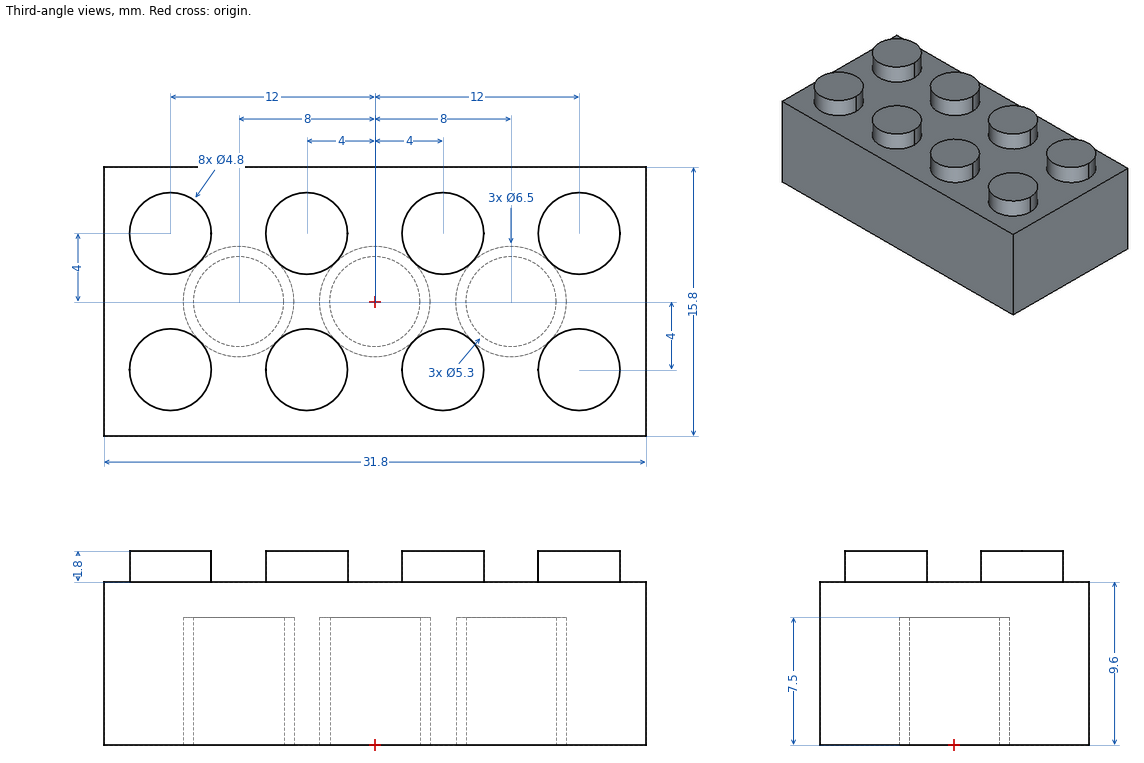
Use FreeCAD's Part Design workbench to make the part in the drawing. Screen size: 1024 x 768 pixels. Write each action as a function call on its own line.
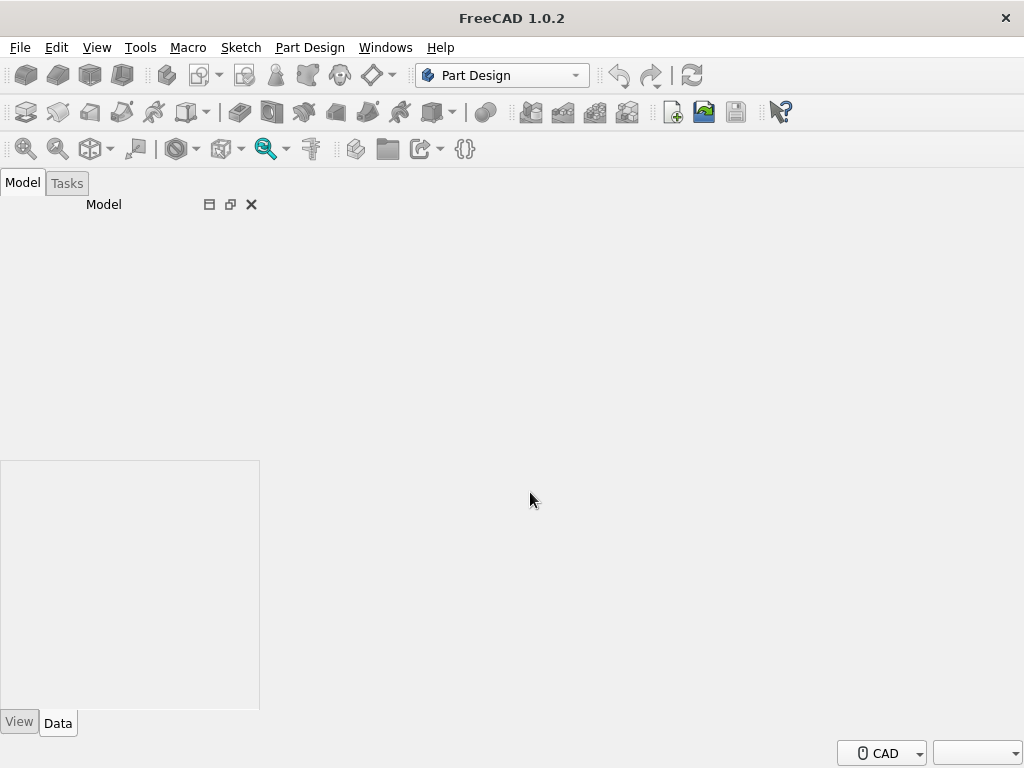
click(672, 112)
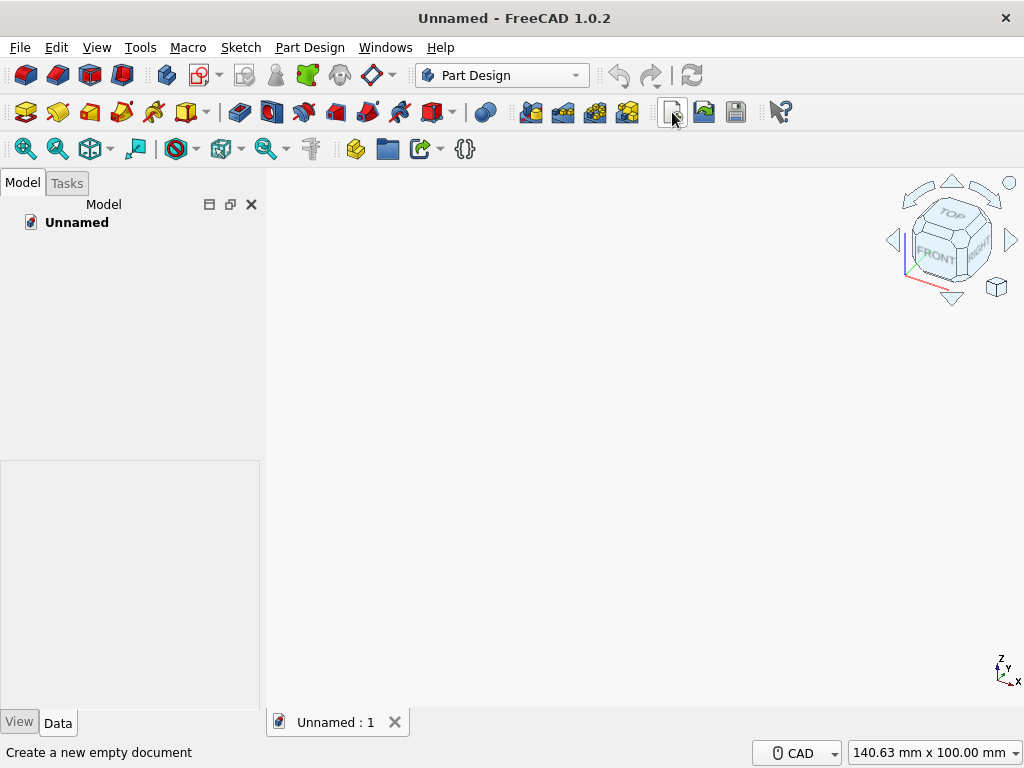
click(200, 76)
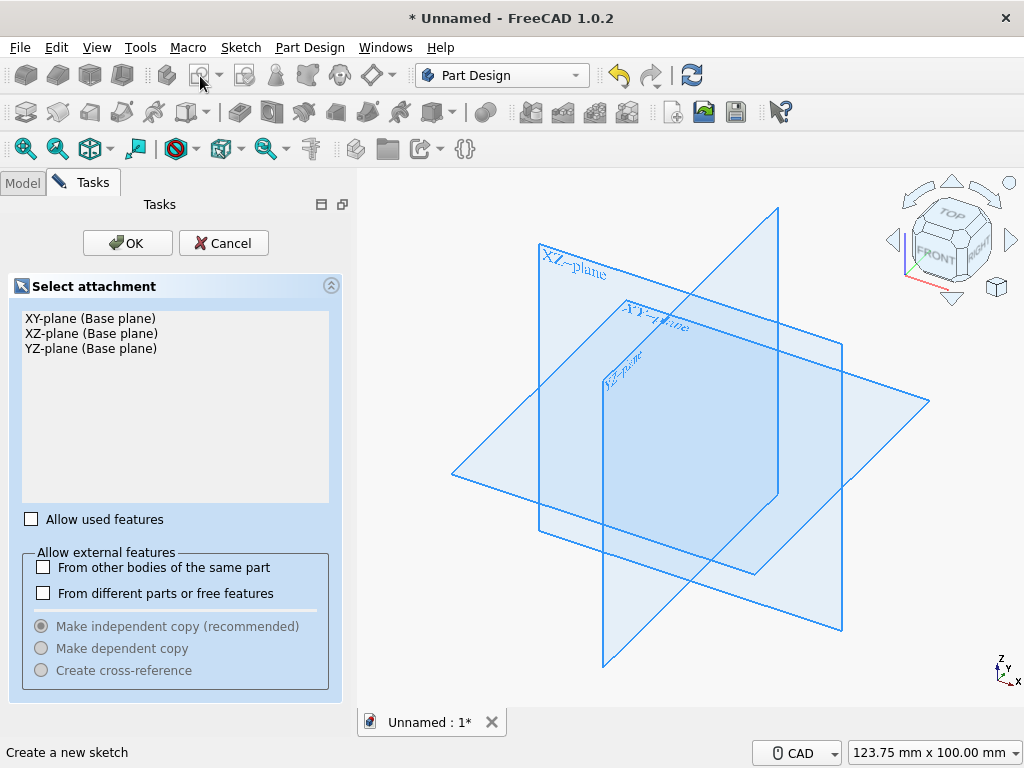
click(82, 318)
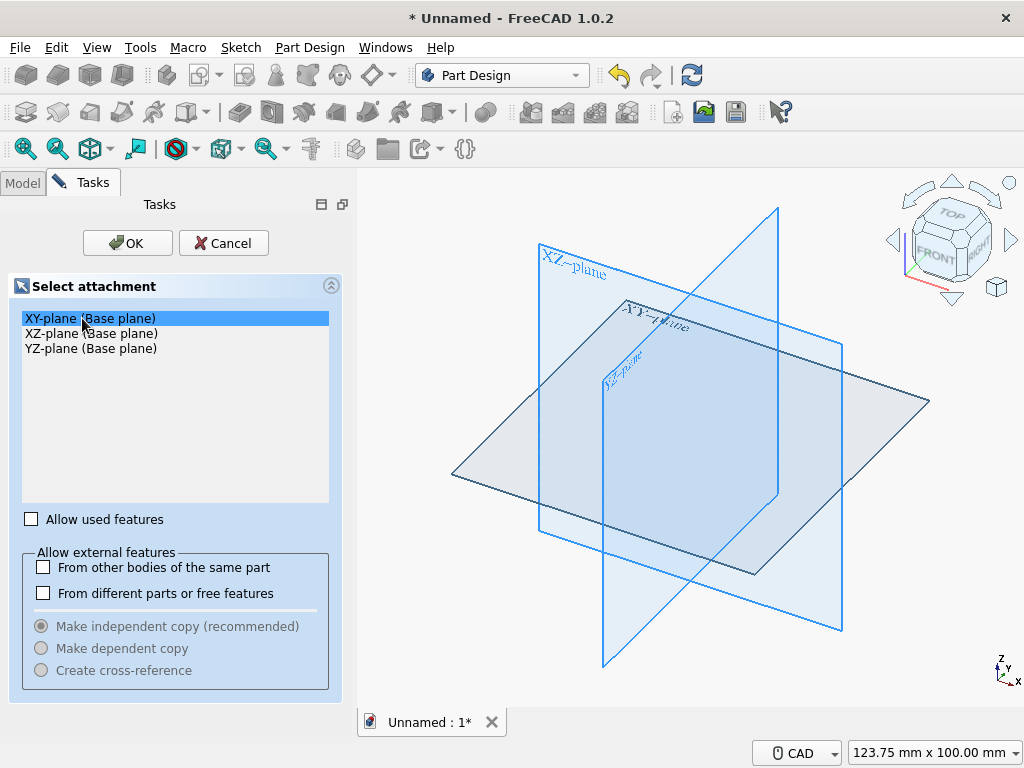
click(128, 243)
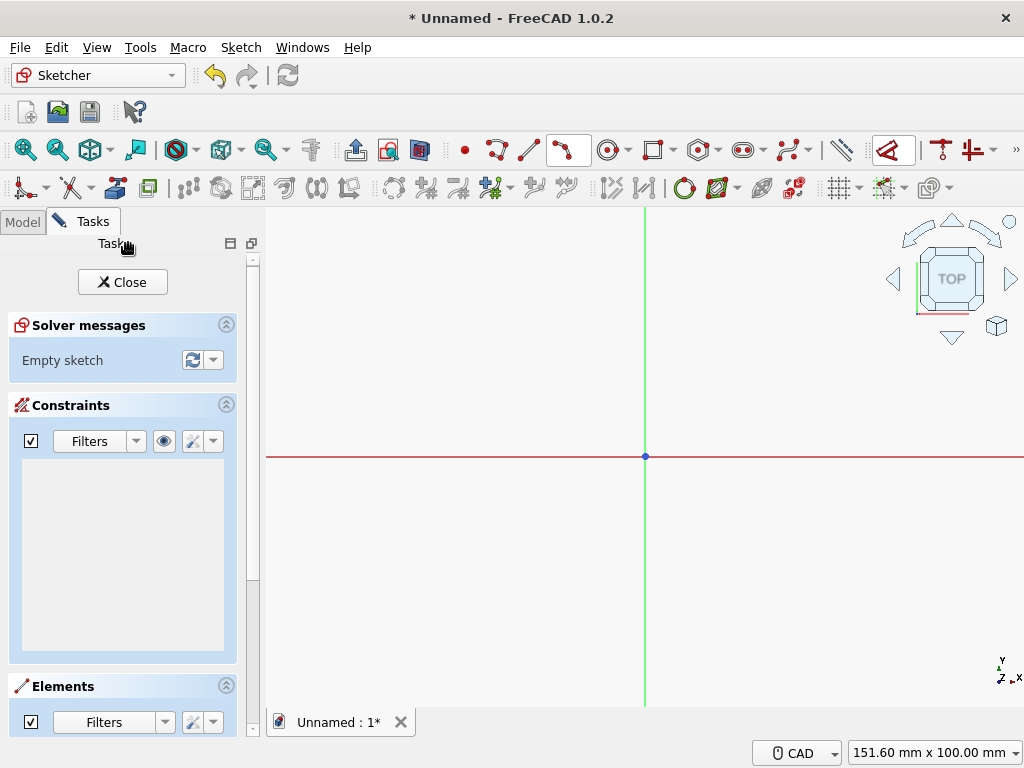
scroll(685, 457, up, 5)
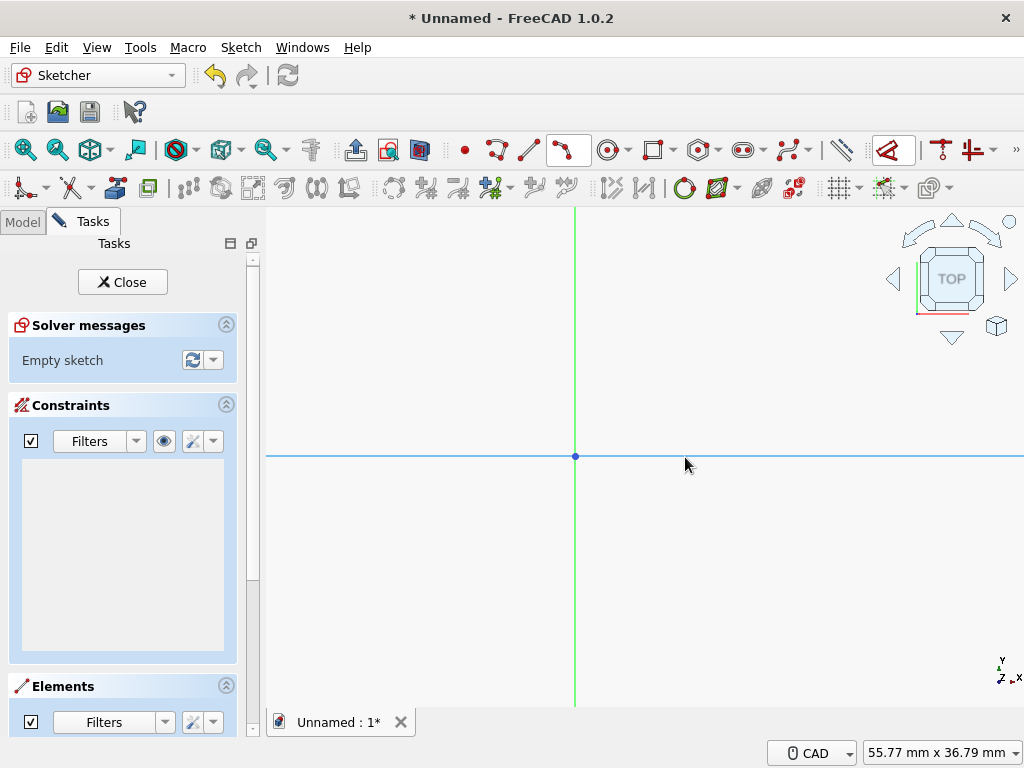
click(676, 150)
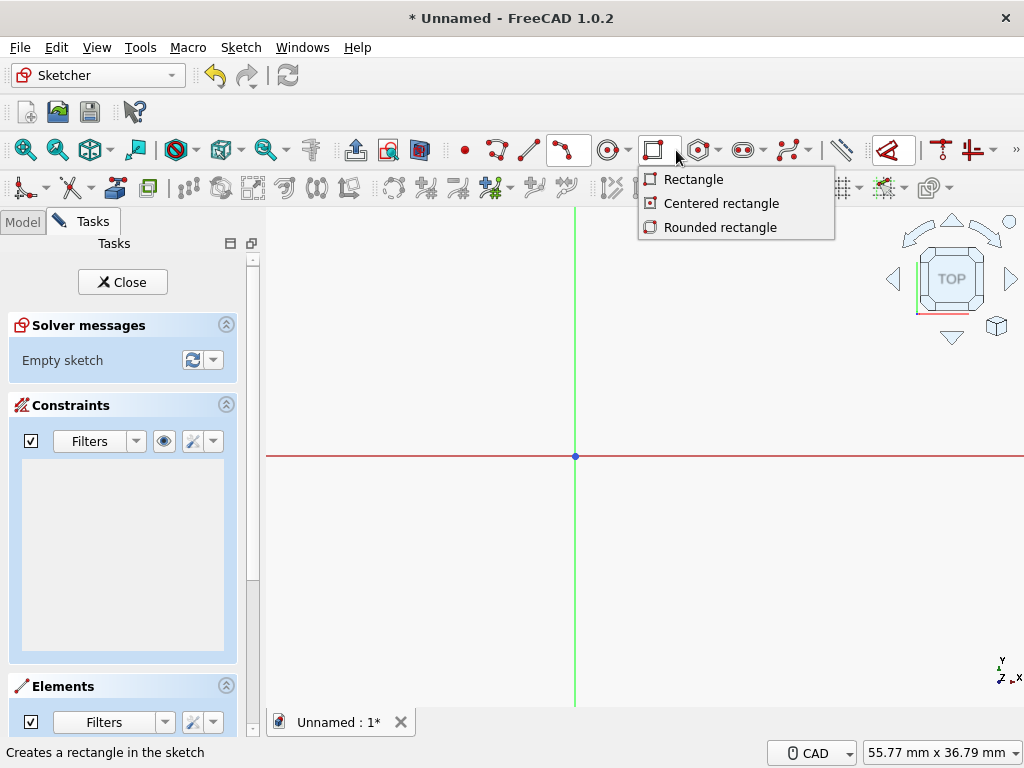
click(736, 203)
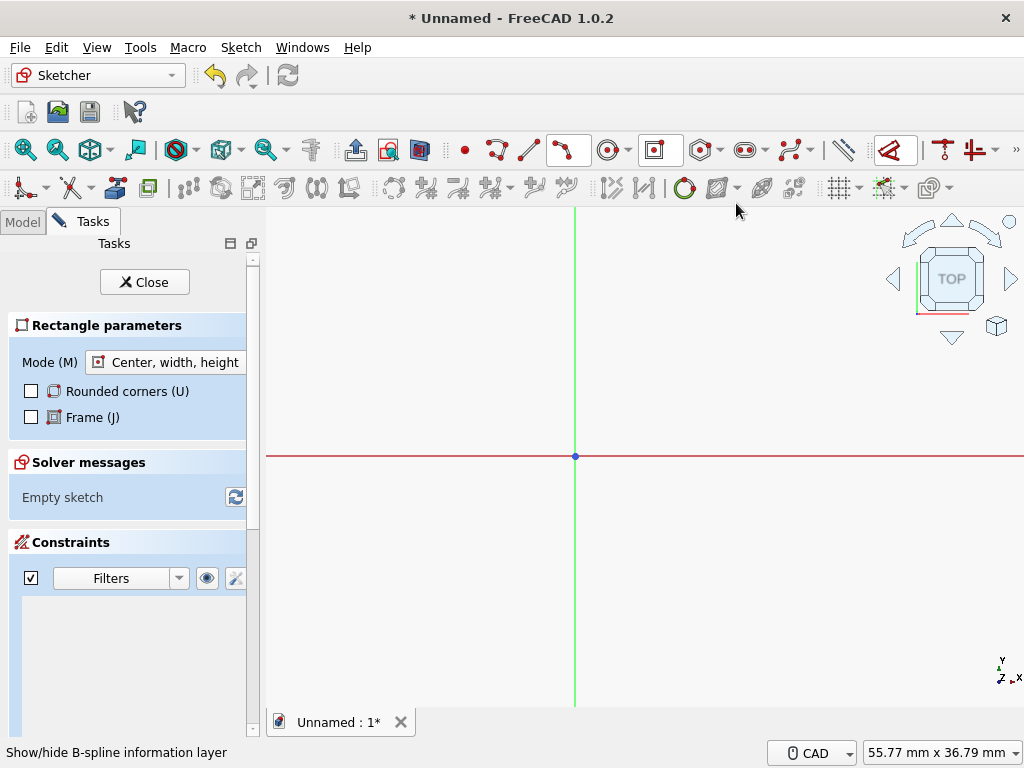
click(575, 456)
move(791, 349)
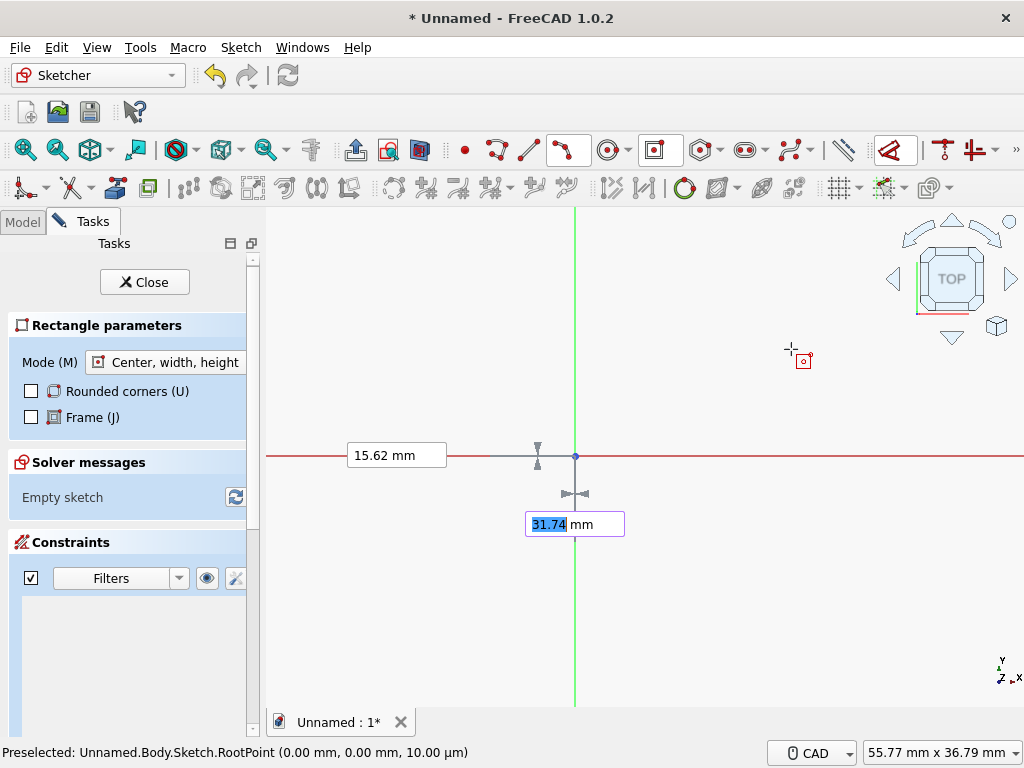
text(31.8)
key(Tab)
text(15.8)
key(Return)
key(Escape)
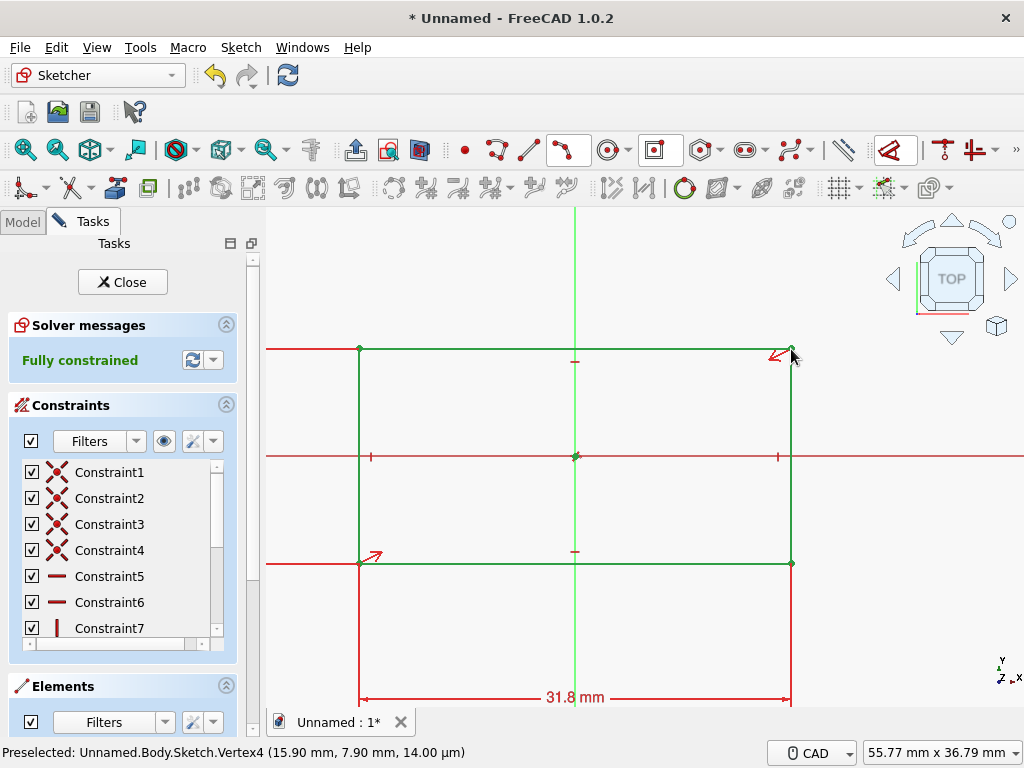
click(123, 282)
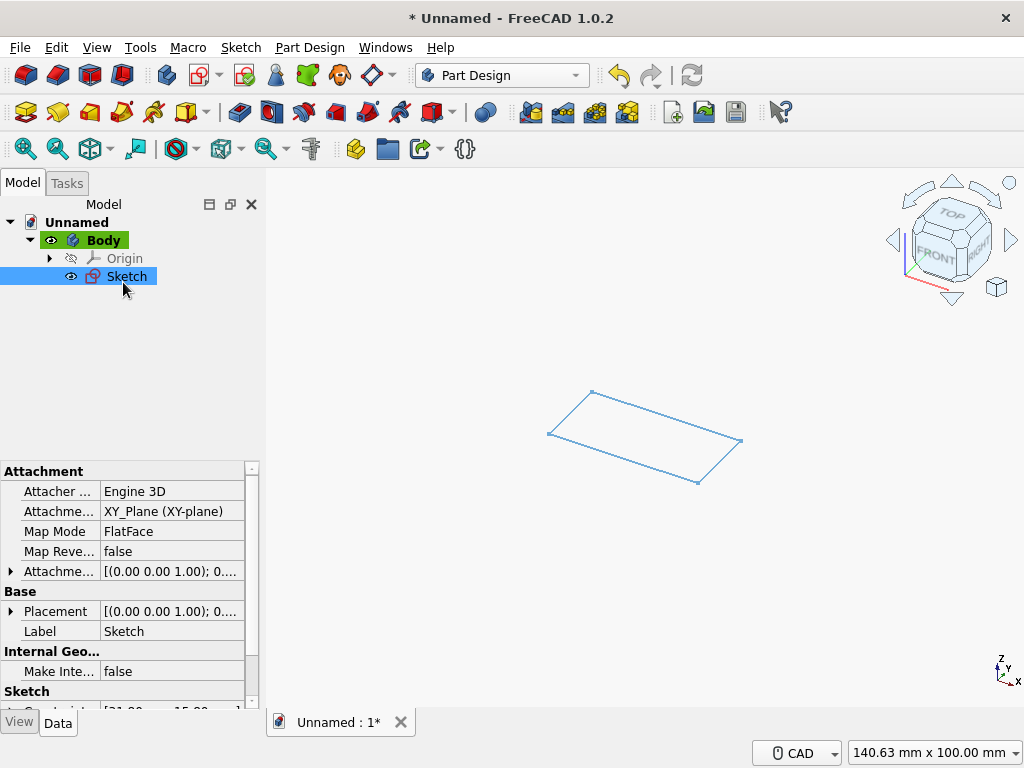
click(26, 112)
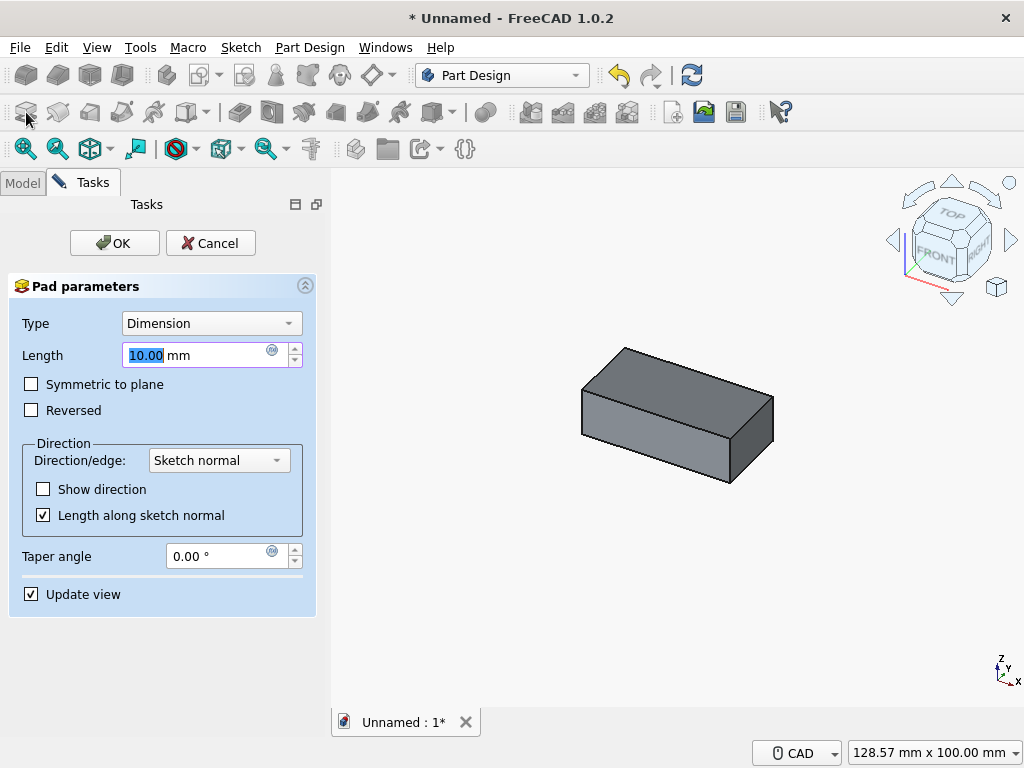
text(9.6)
key(Tab)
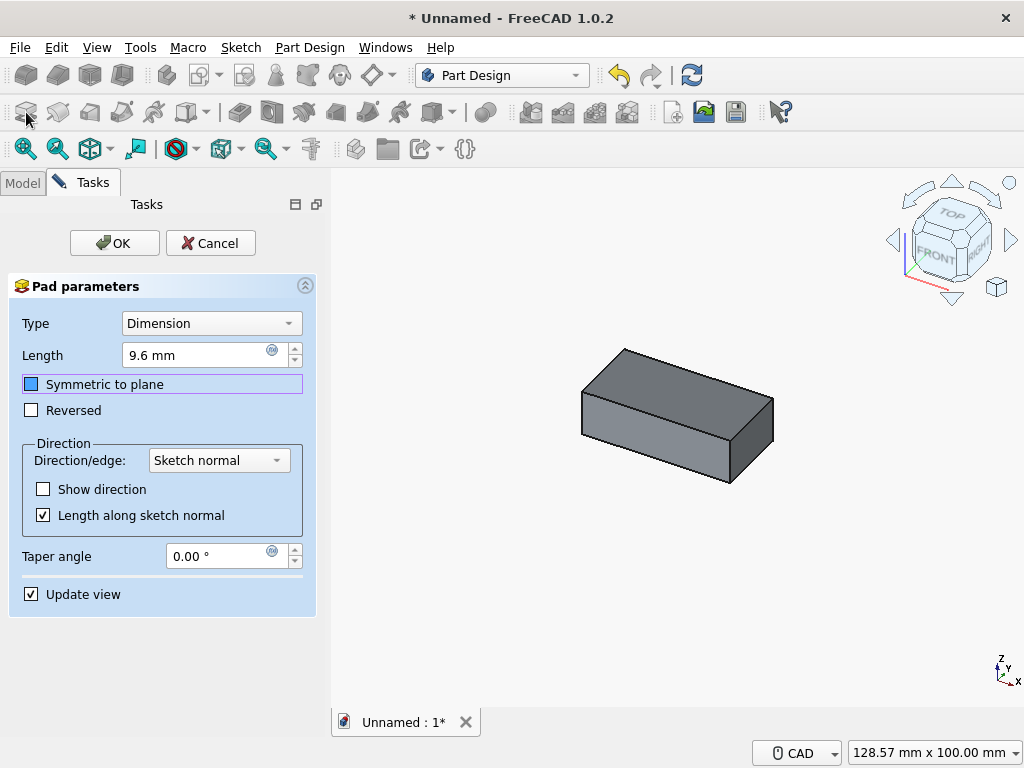
click(115, 243)